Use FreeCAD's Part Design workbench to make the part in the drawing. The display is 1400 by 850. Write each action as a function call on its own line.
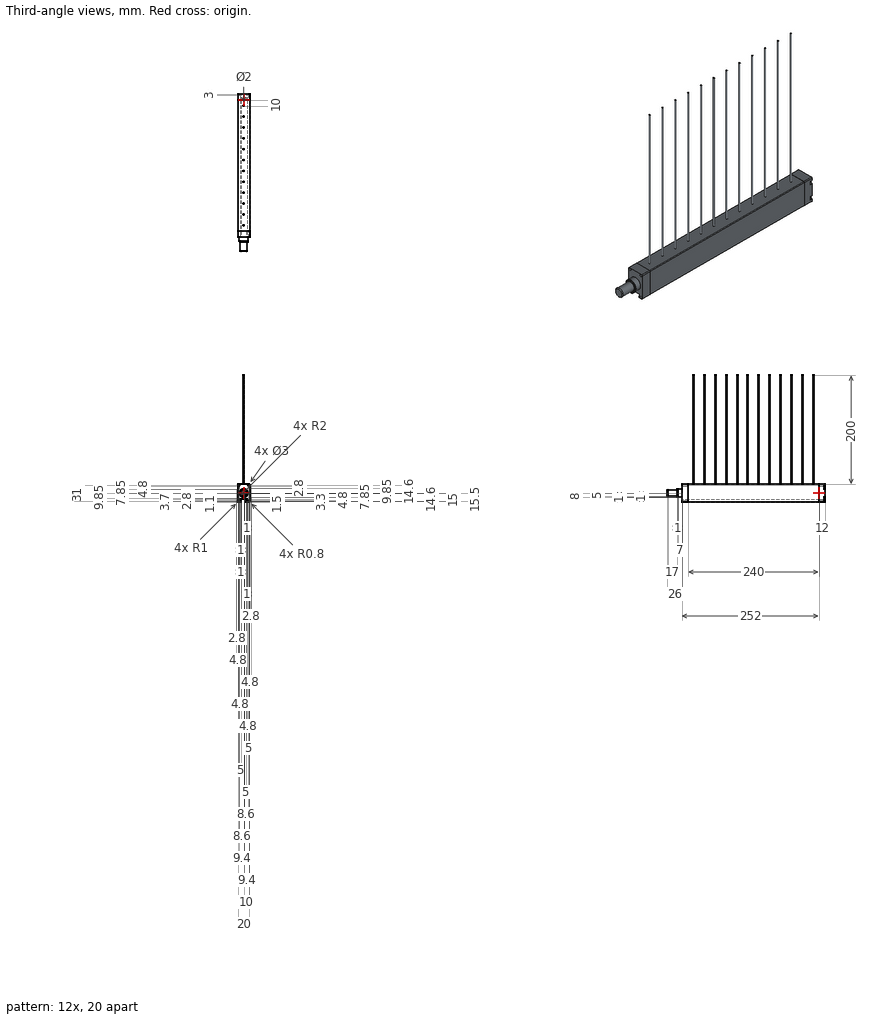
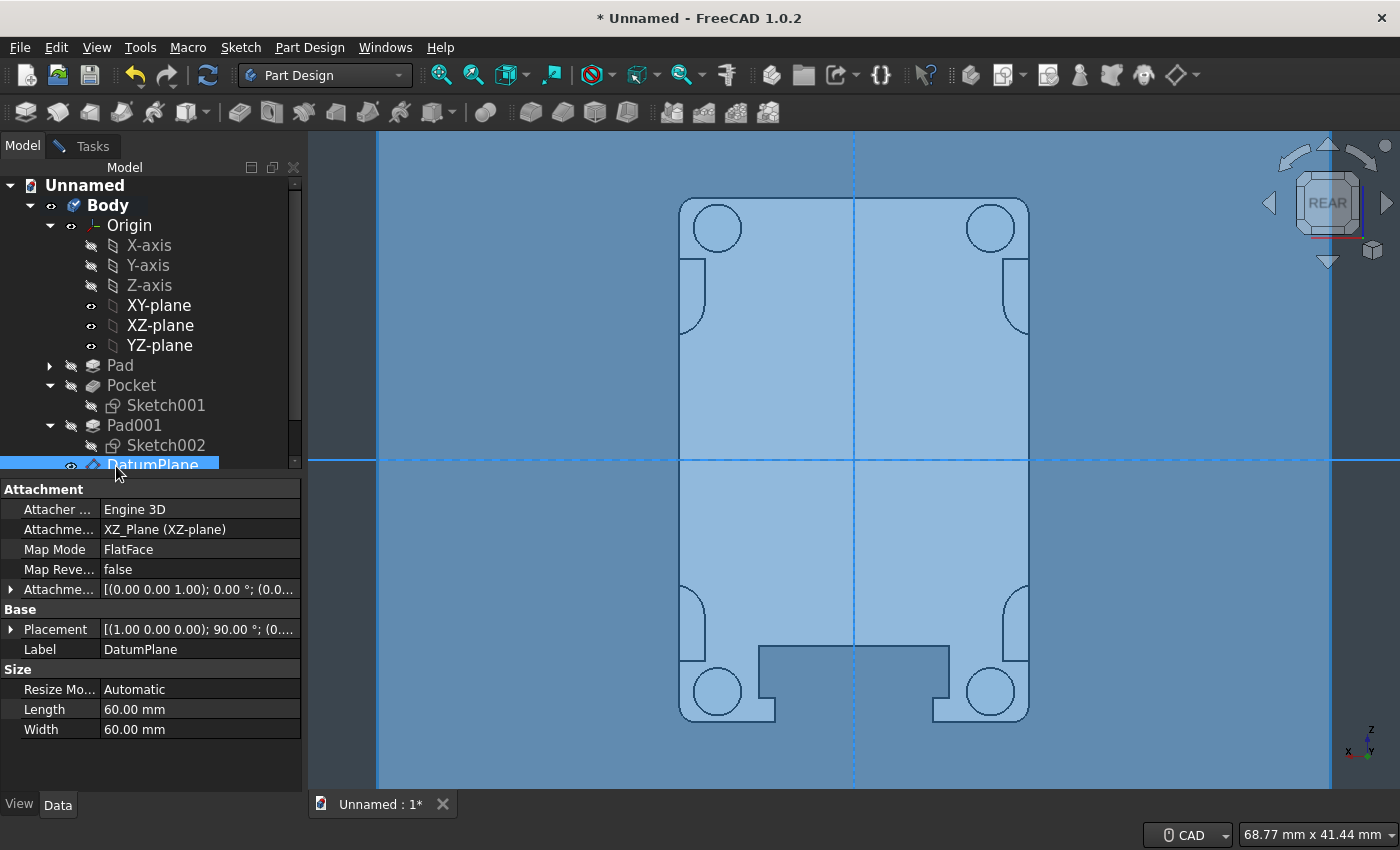
click(84, 145)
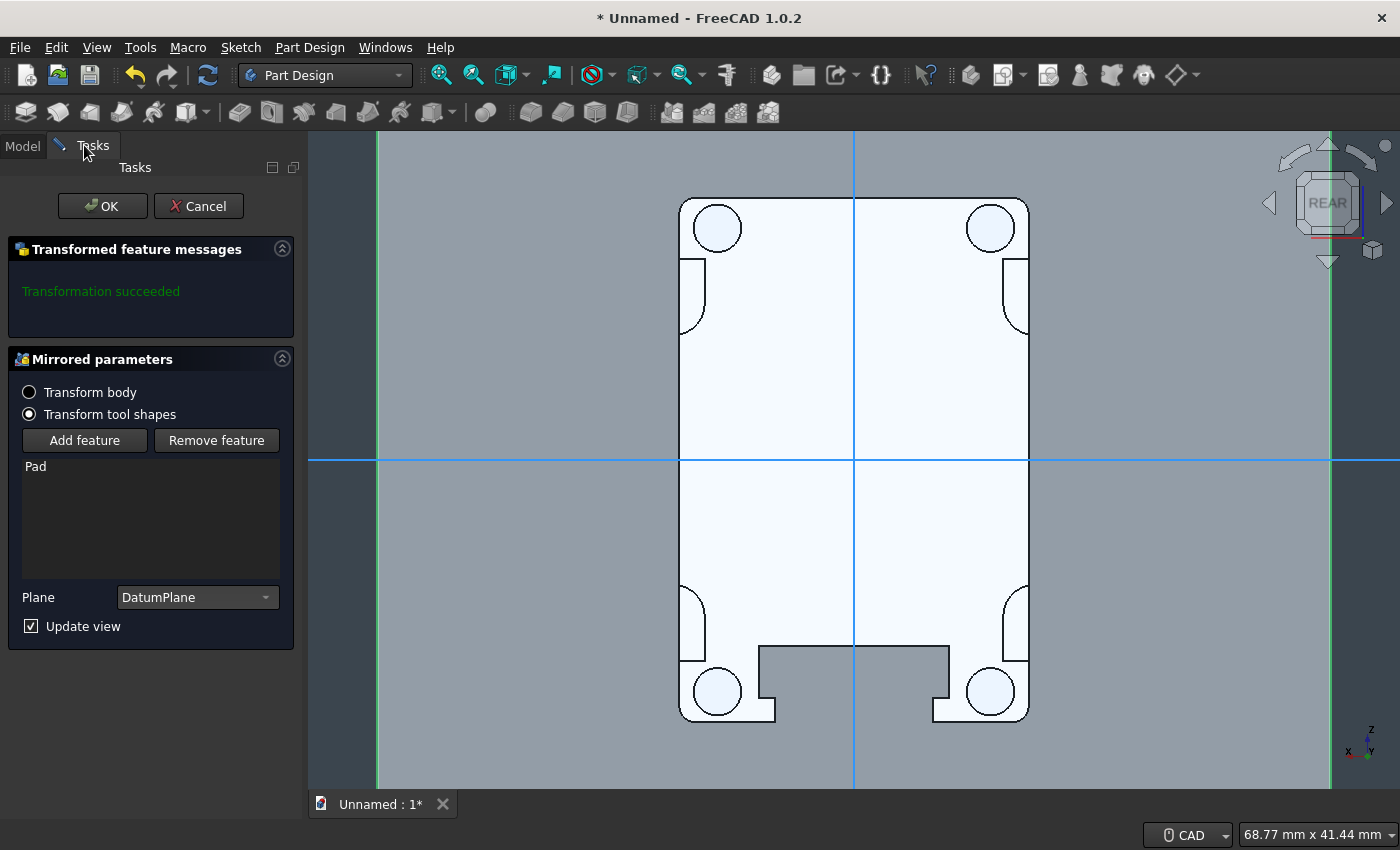
click(103, 206)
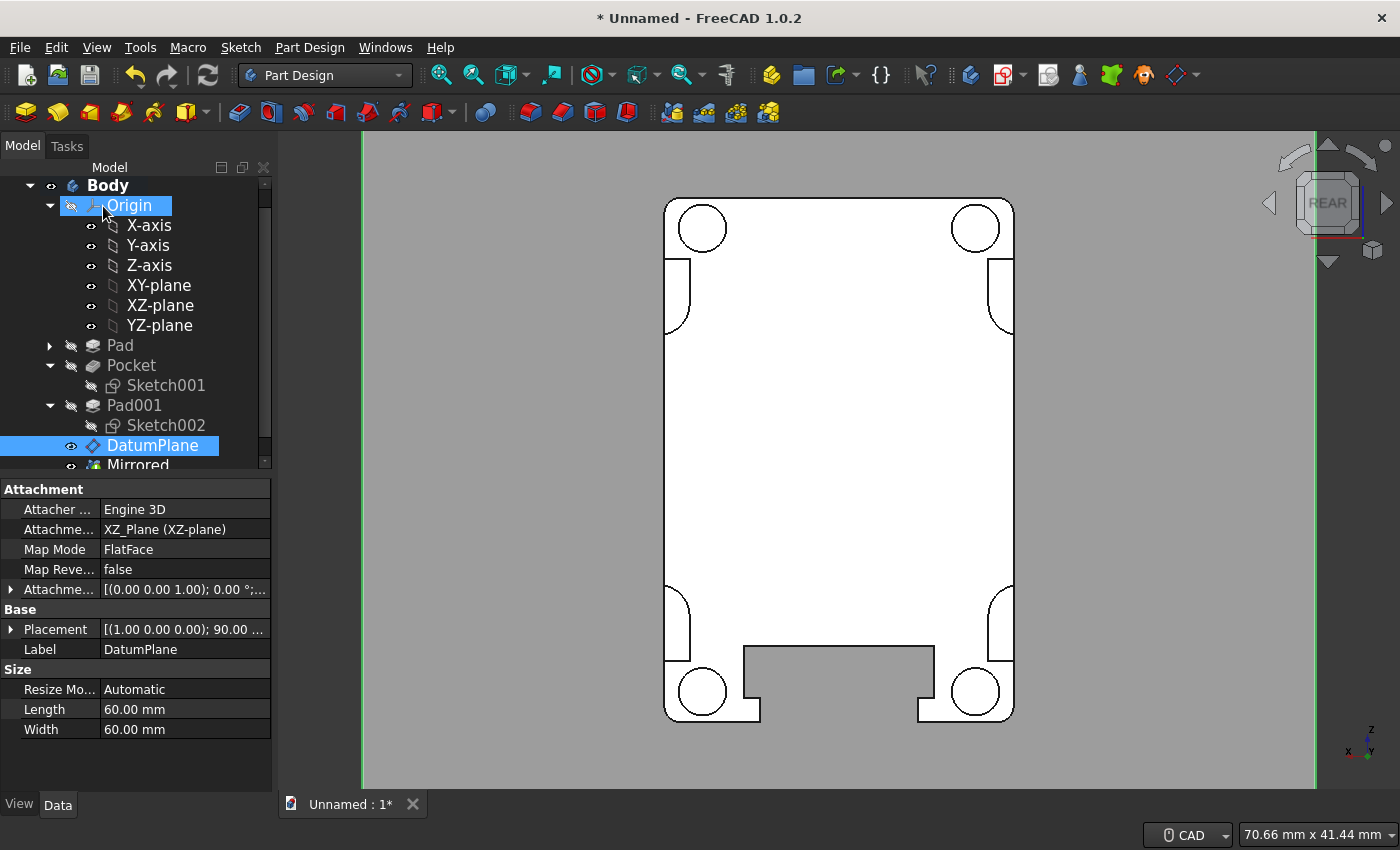
click(116, 446)
key(space)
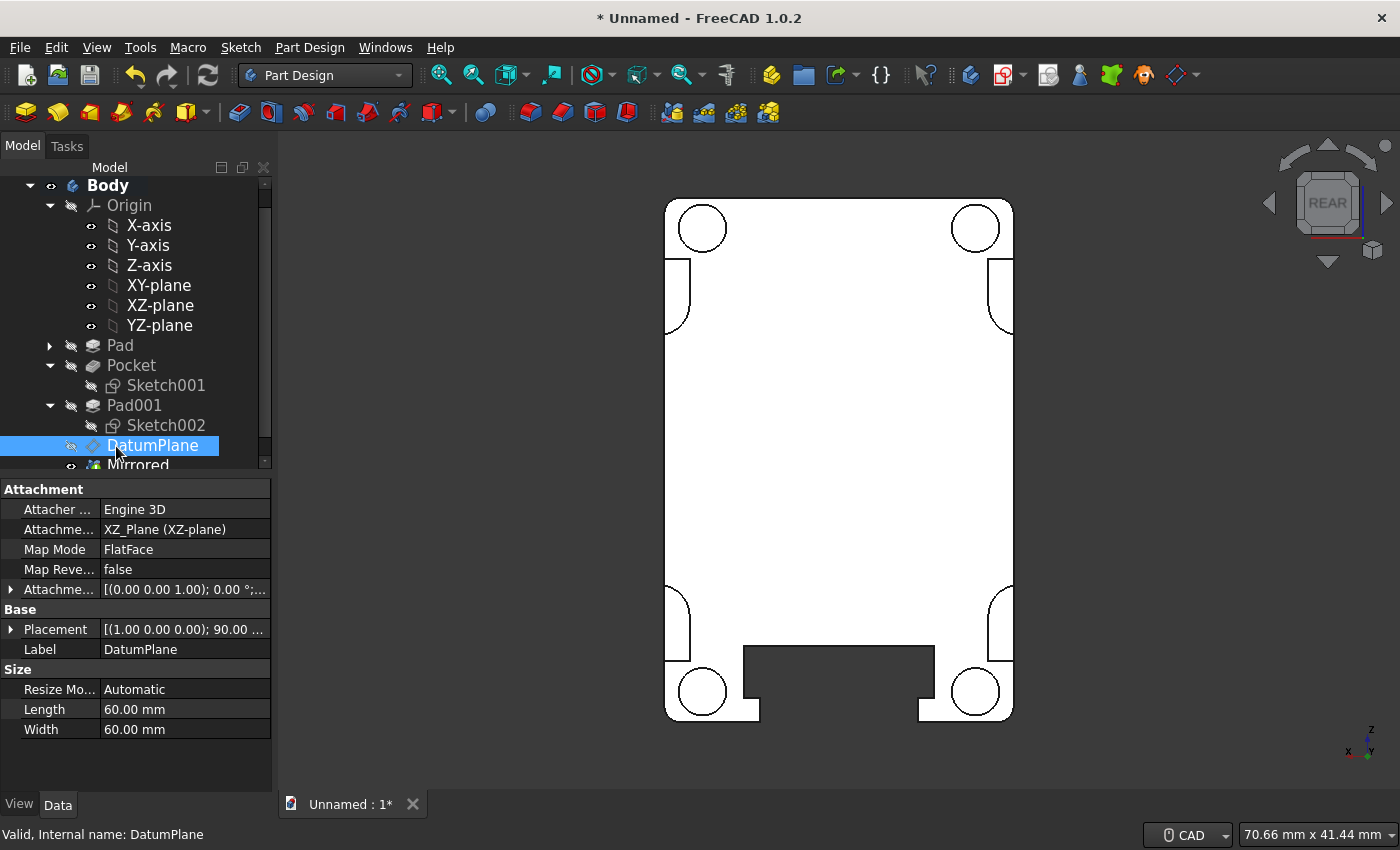
click(318, 749)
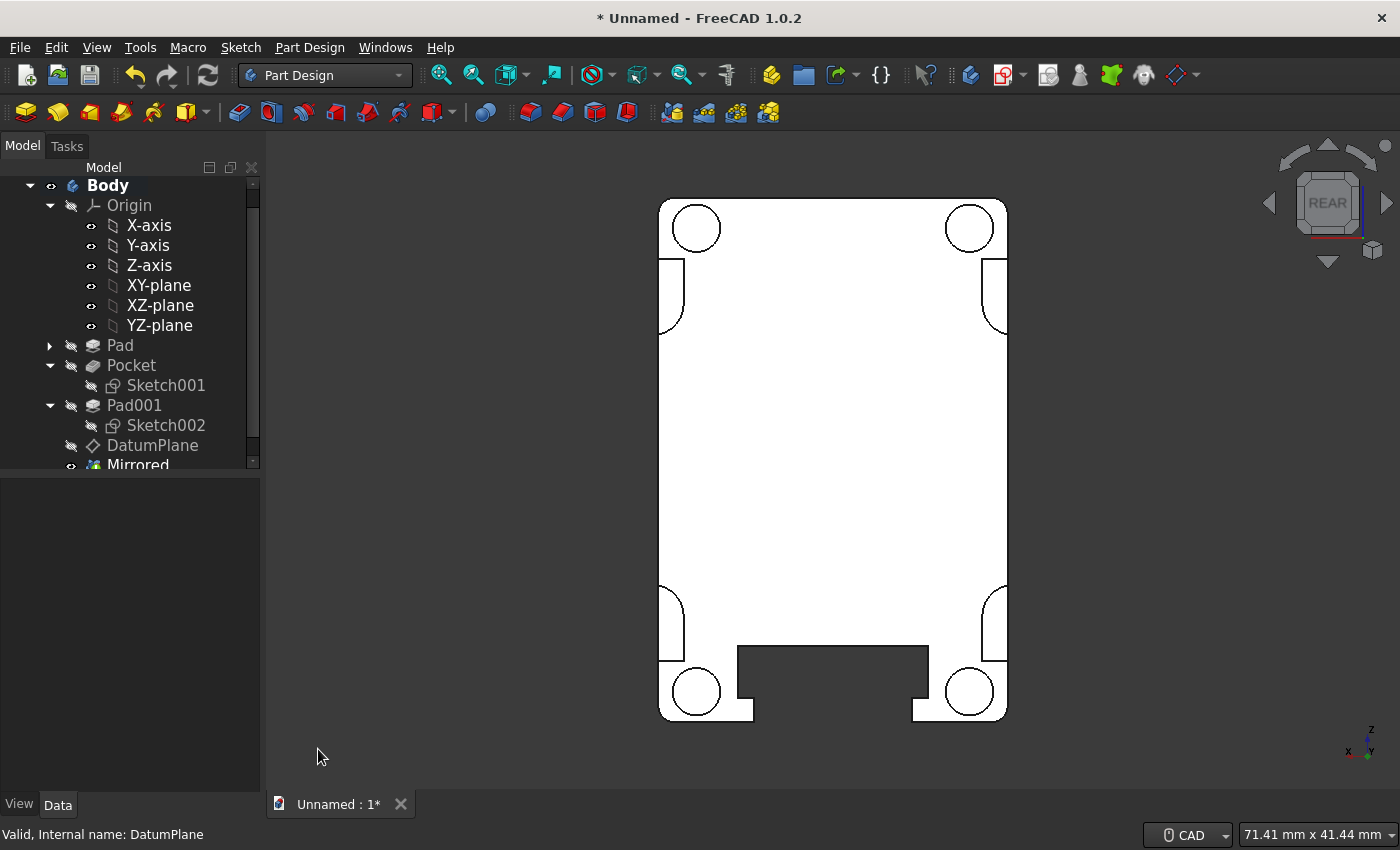
click(1004, 76)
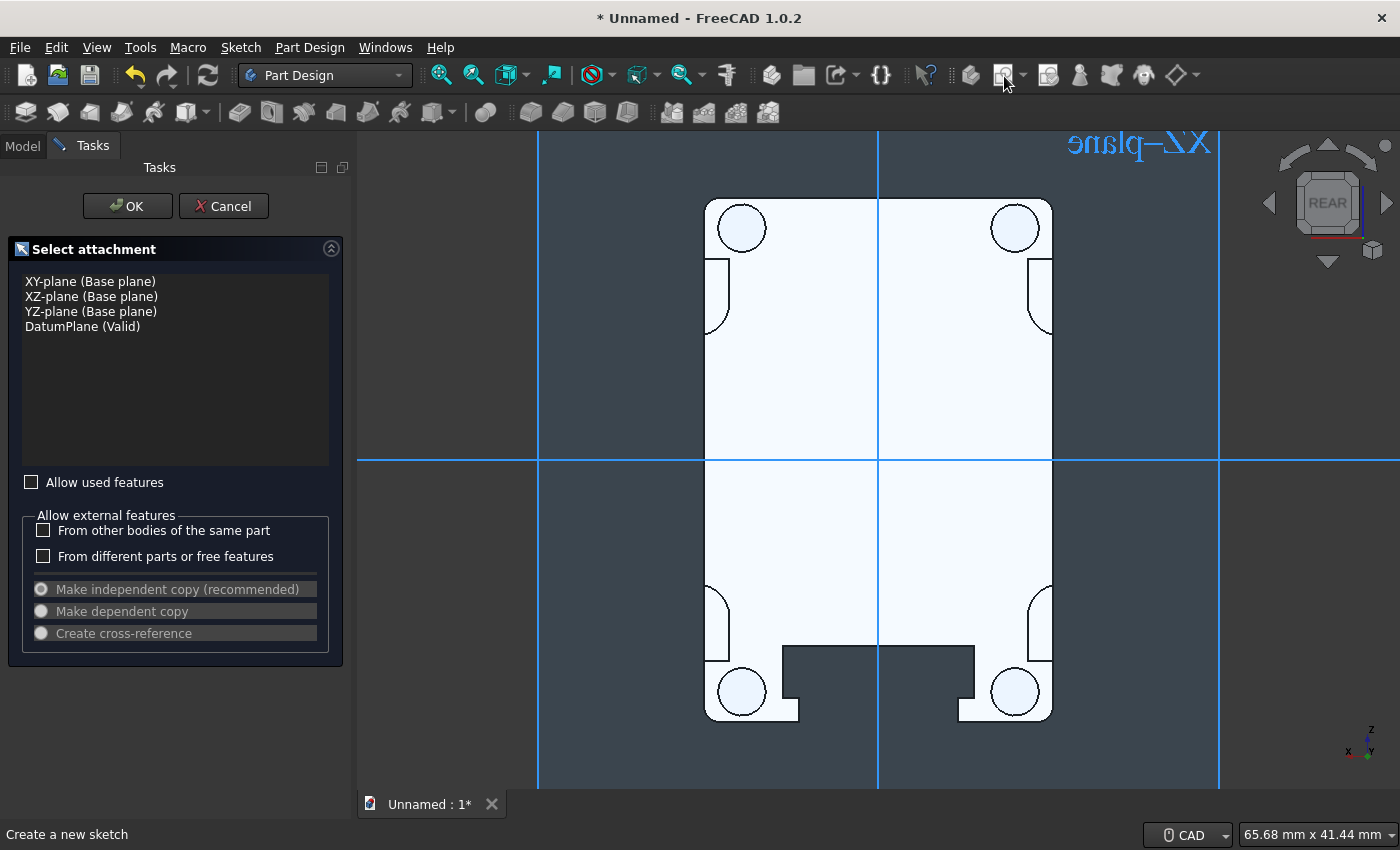
click(82, 312)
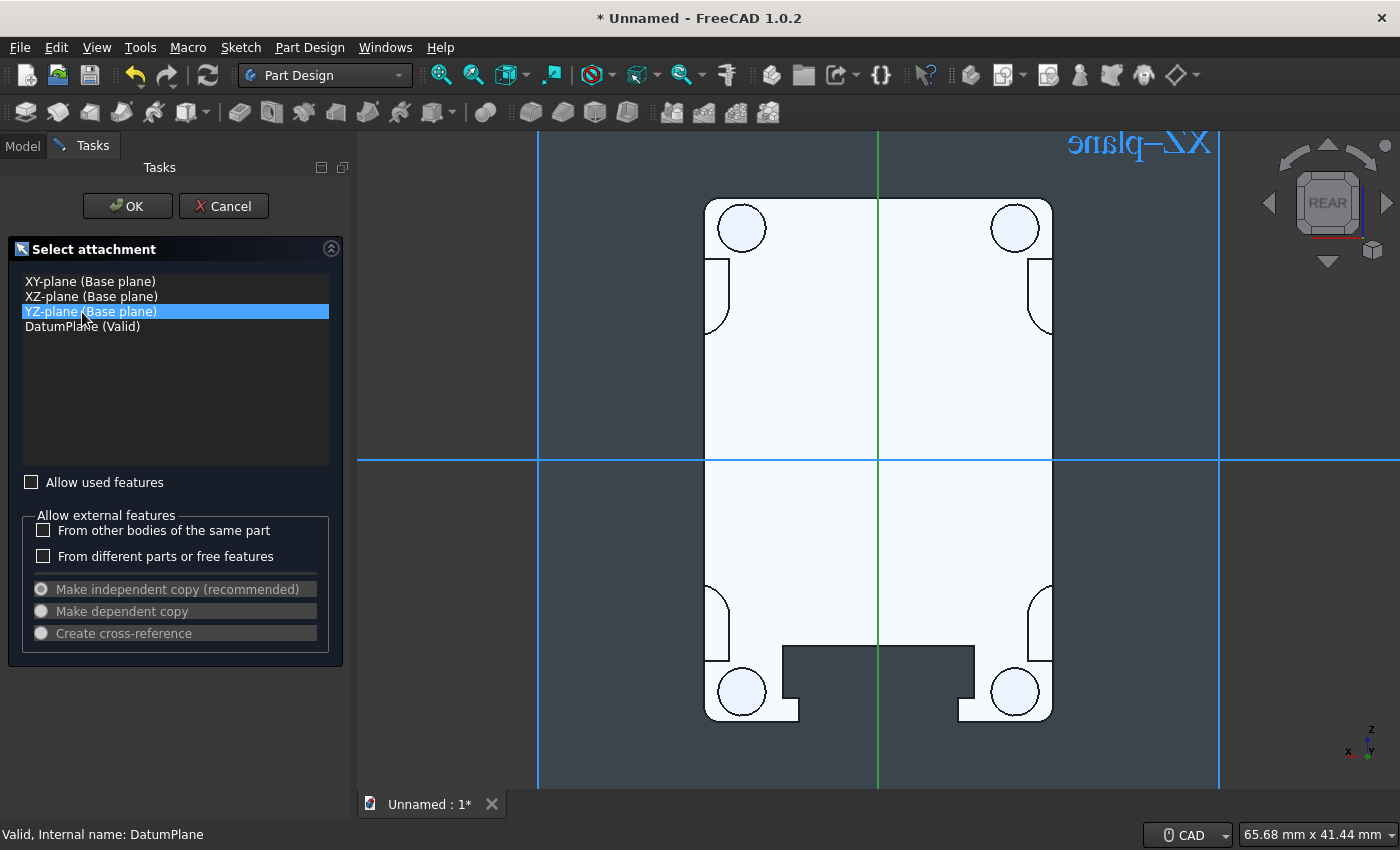
click(128, 206)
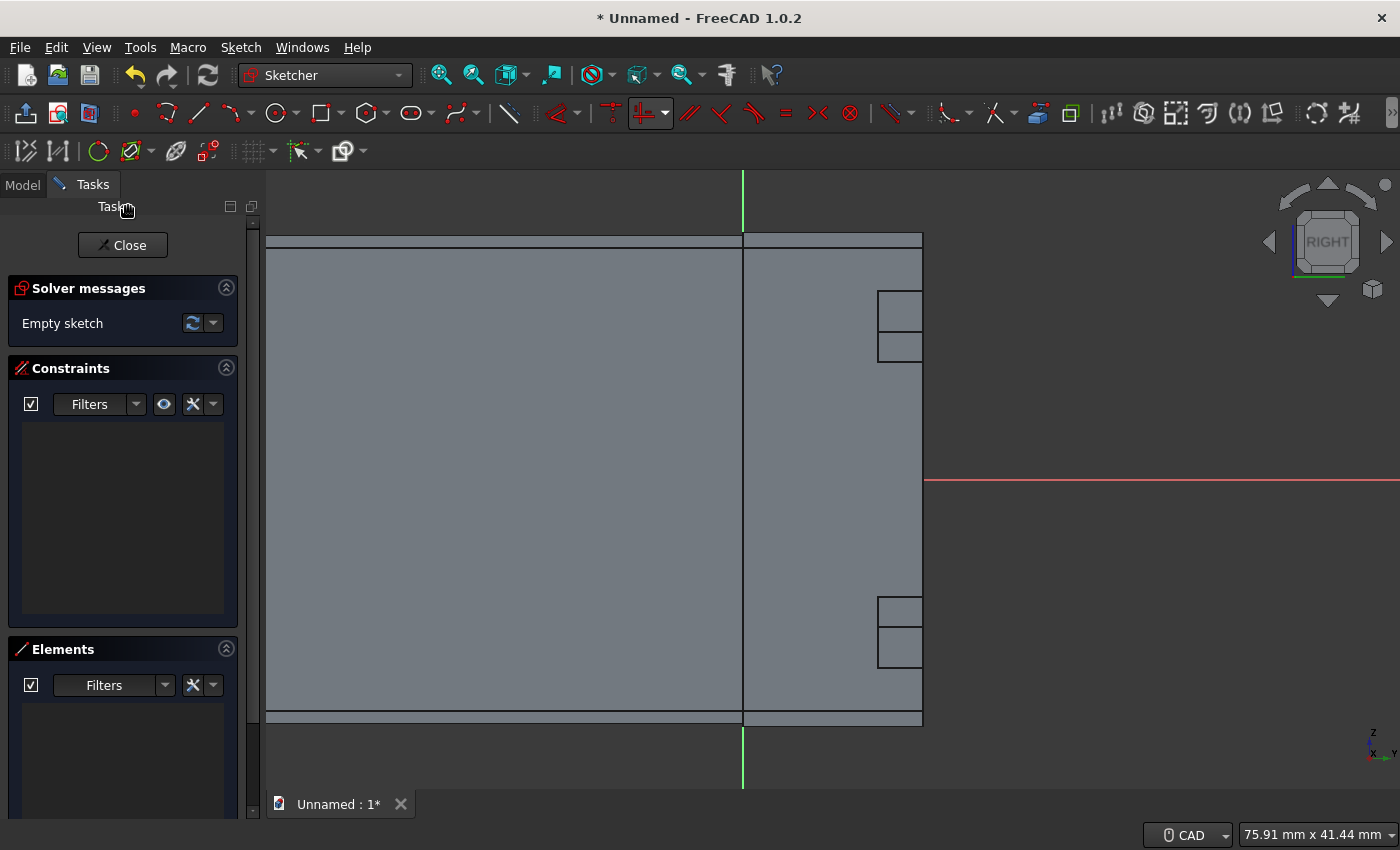
click(90, 114)